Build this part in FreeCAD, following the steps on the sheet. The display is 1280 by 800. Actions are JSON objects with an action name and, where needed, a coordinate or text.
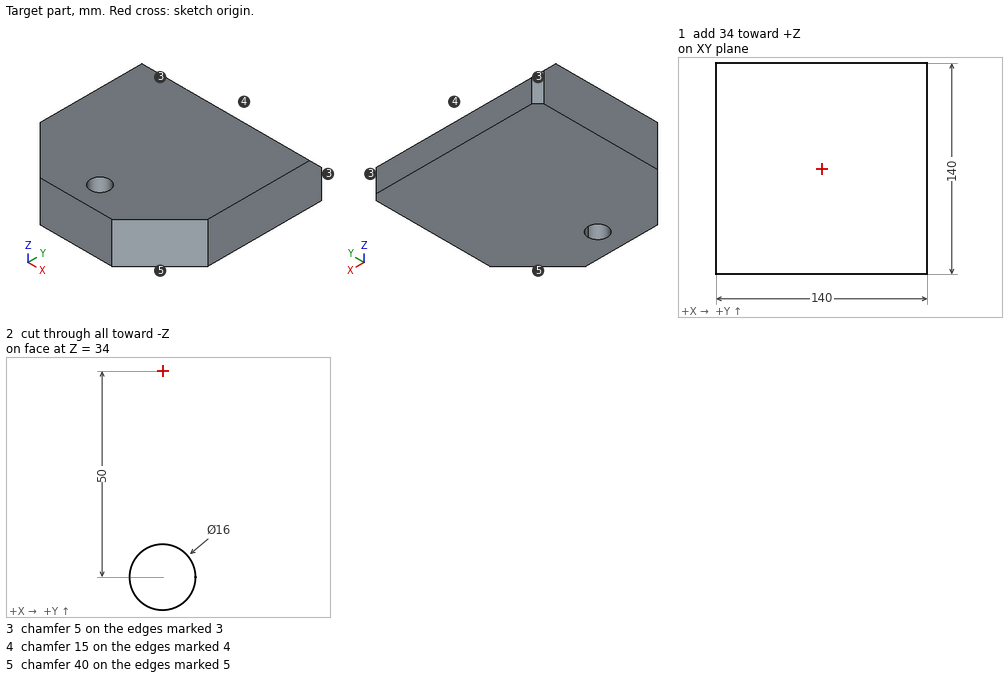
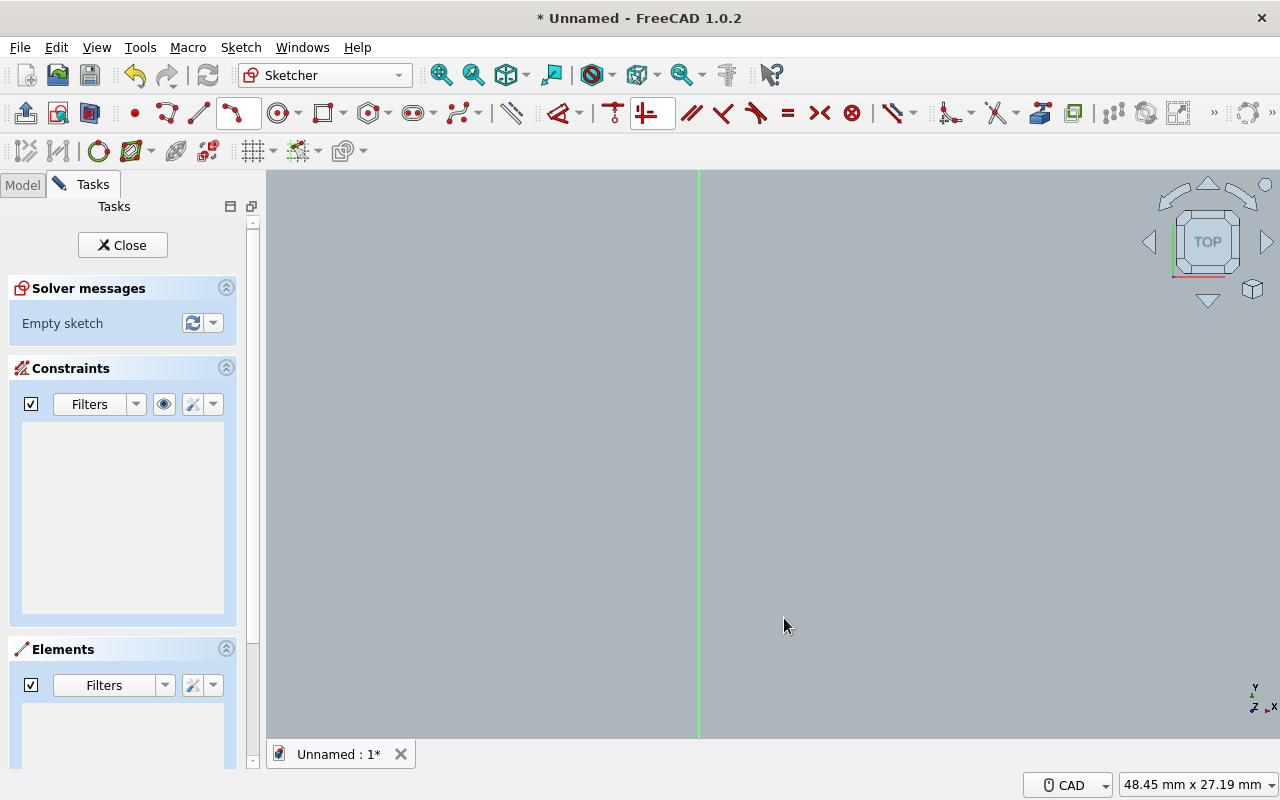
{"action": "left_click", "coordinate": [278, 114]}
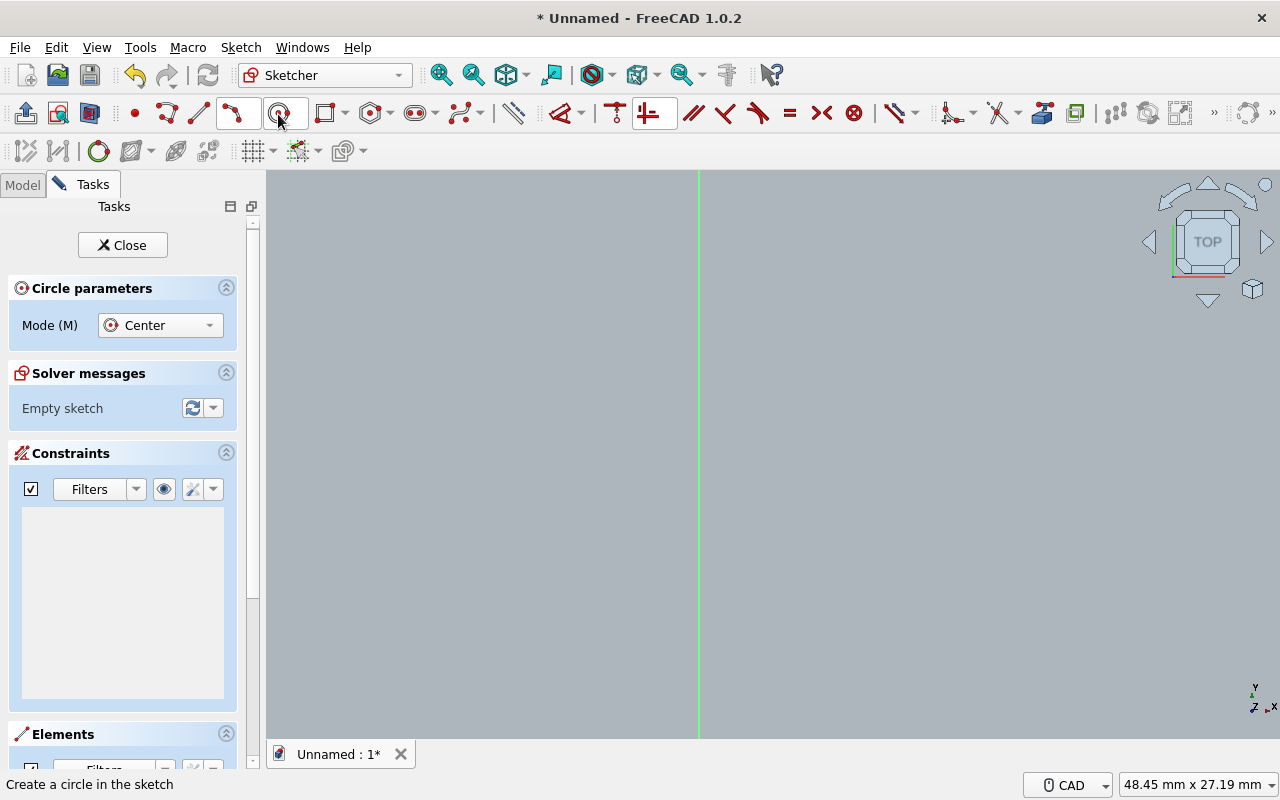
{"action": "left_click", "coordinate": [699, 451]}
{"action": "left_click", "coordinate": [818, 333]}
{"action": "key", "text": "Escape"}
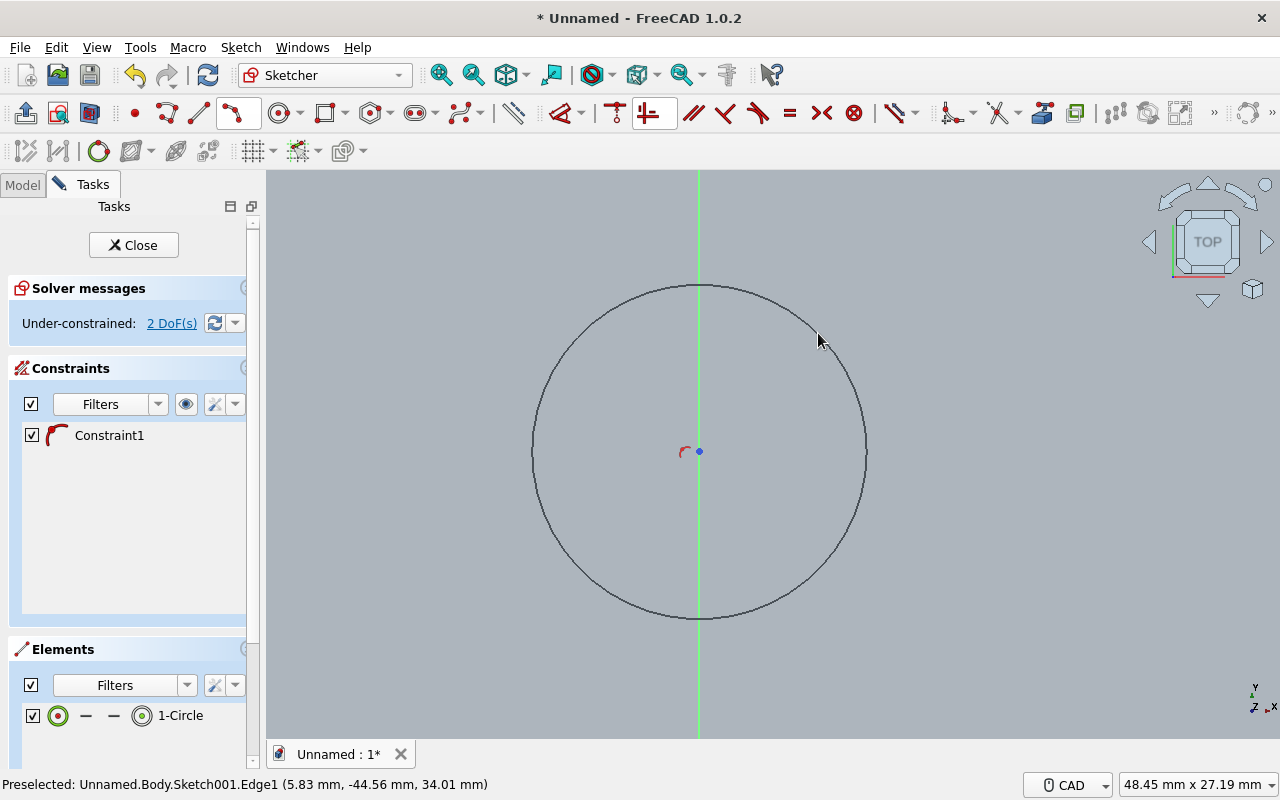
{"action": "left_click", "coordinate": [560, 114]}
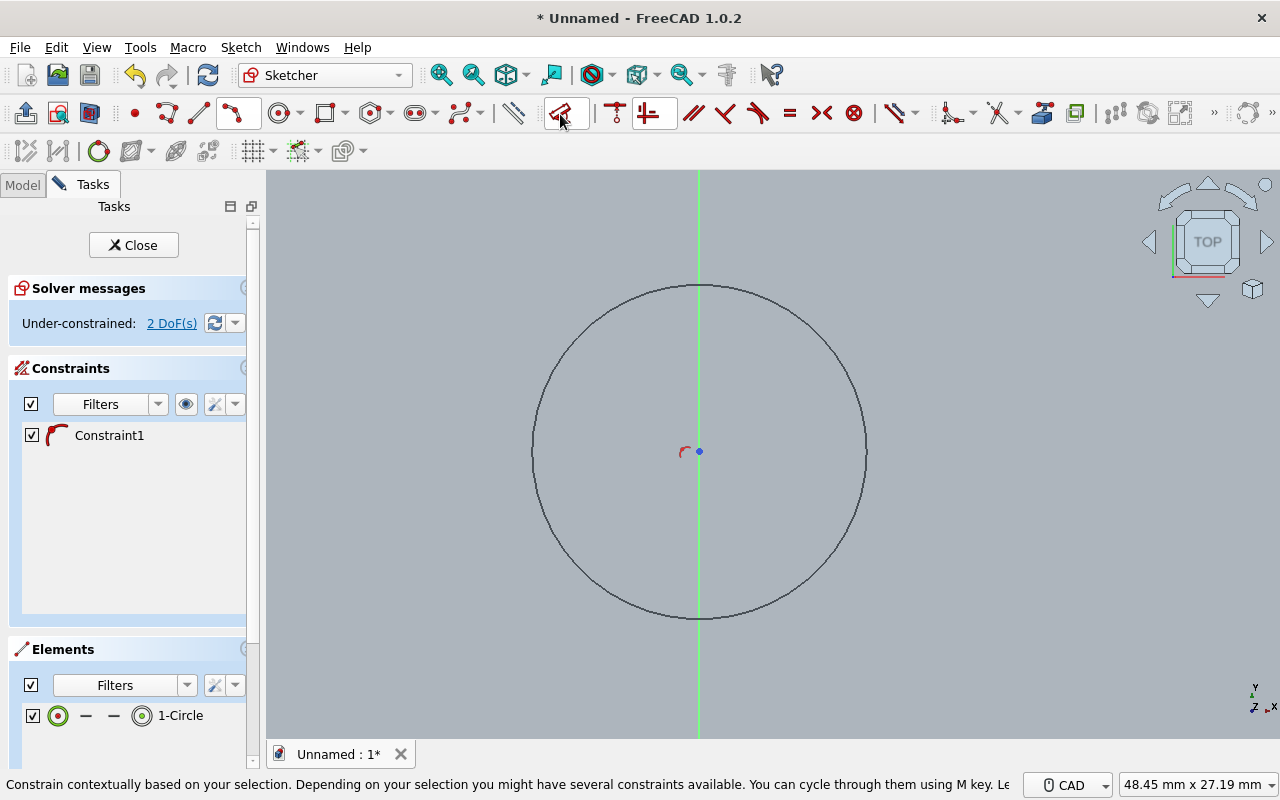
{"action": "left_click", "coordinate": [817, 333]}
{"action": "left_click", "coordinate": [839, 310]}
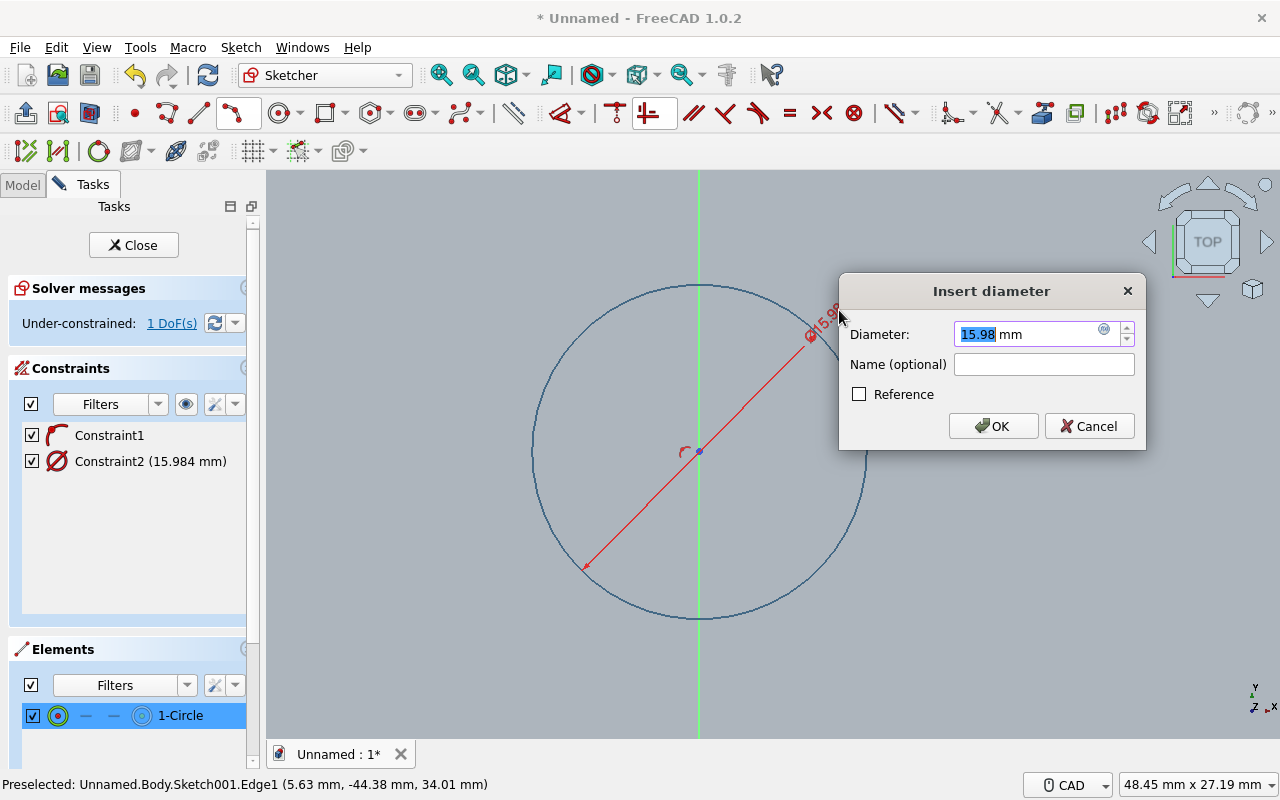
{"action": "type", "text": "16"}
{"action": "key", "text": "Return"}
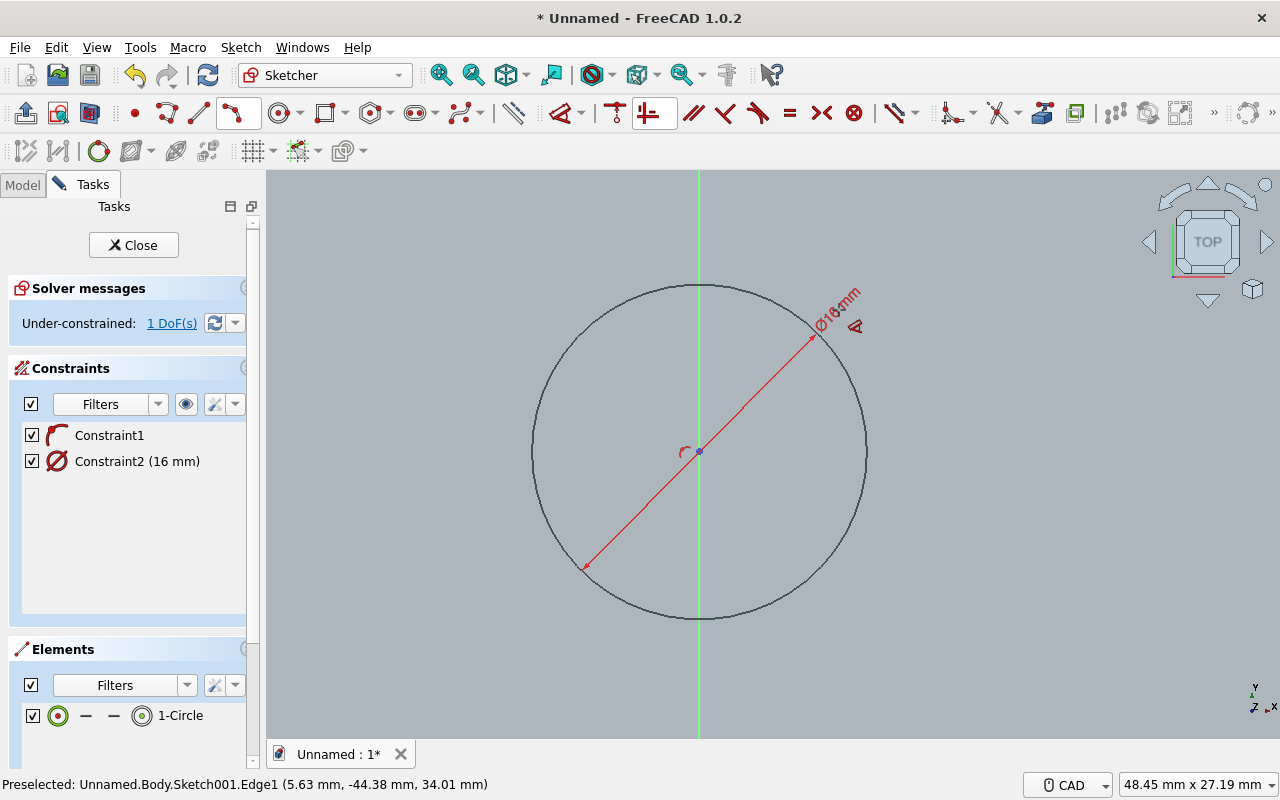
{"action": "left_click", "coordinate": [699, 452]}
{"action": "left_click", "coordinate": [733, 325]}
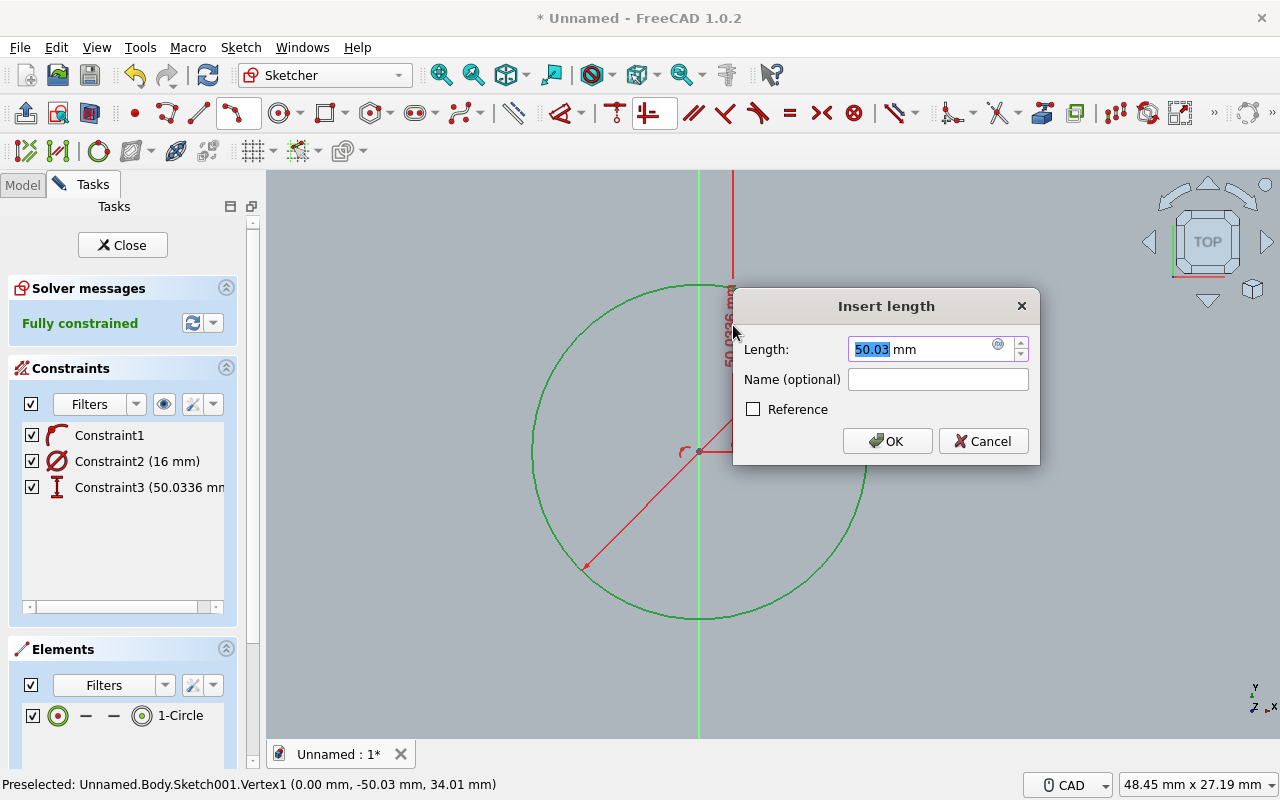
{"action": "type", "text": "50"}
{"action": "key", "text": "Return"}
{"action": "key", "text": "Escape"}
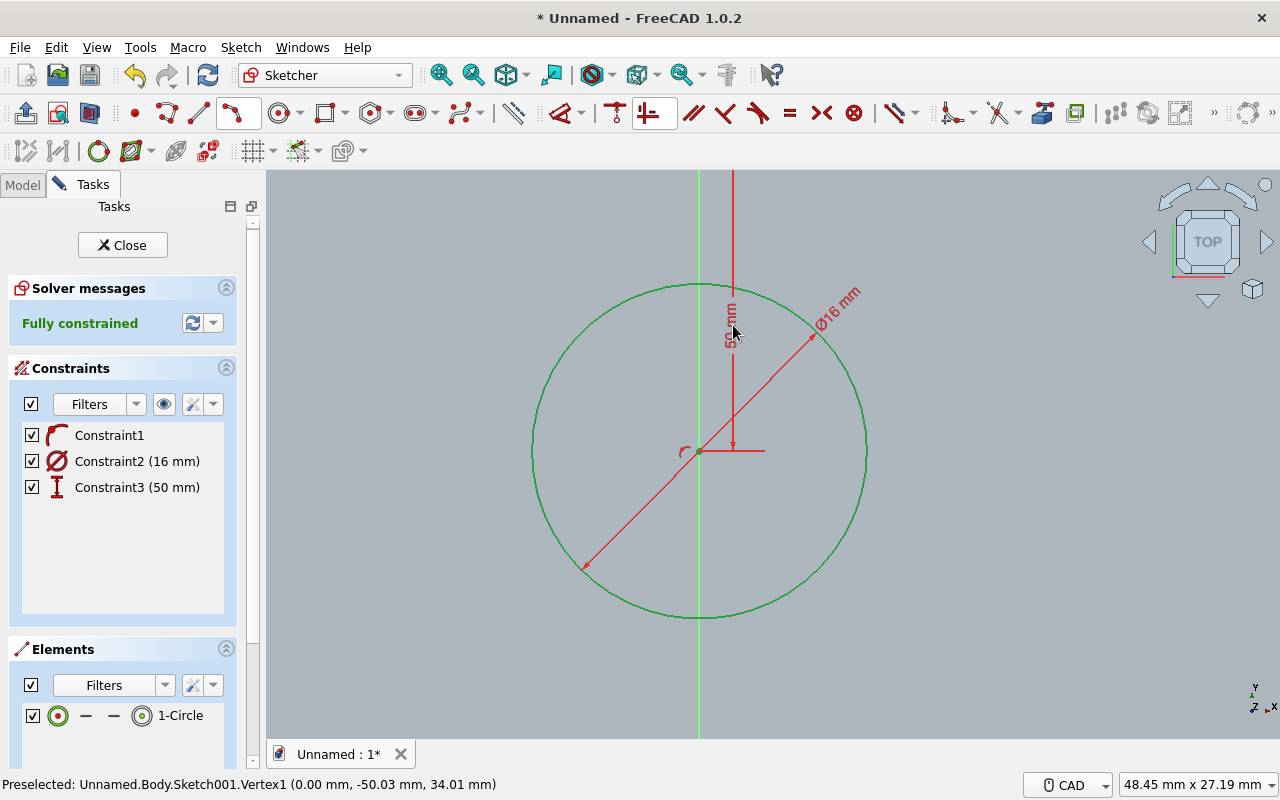
{"action": "left_click", "coordinate": [123, 245]}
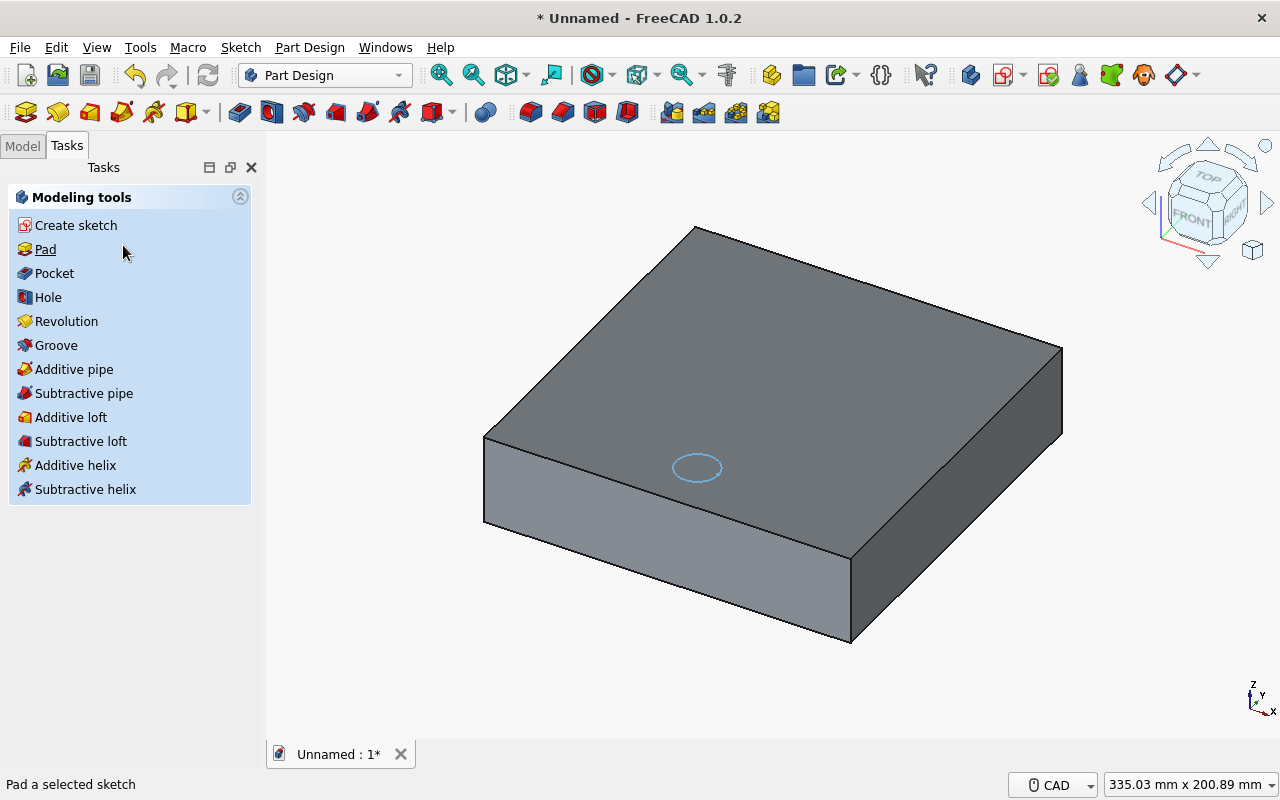
{"action": "left_click", "coordinate": [240, 112]}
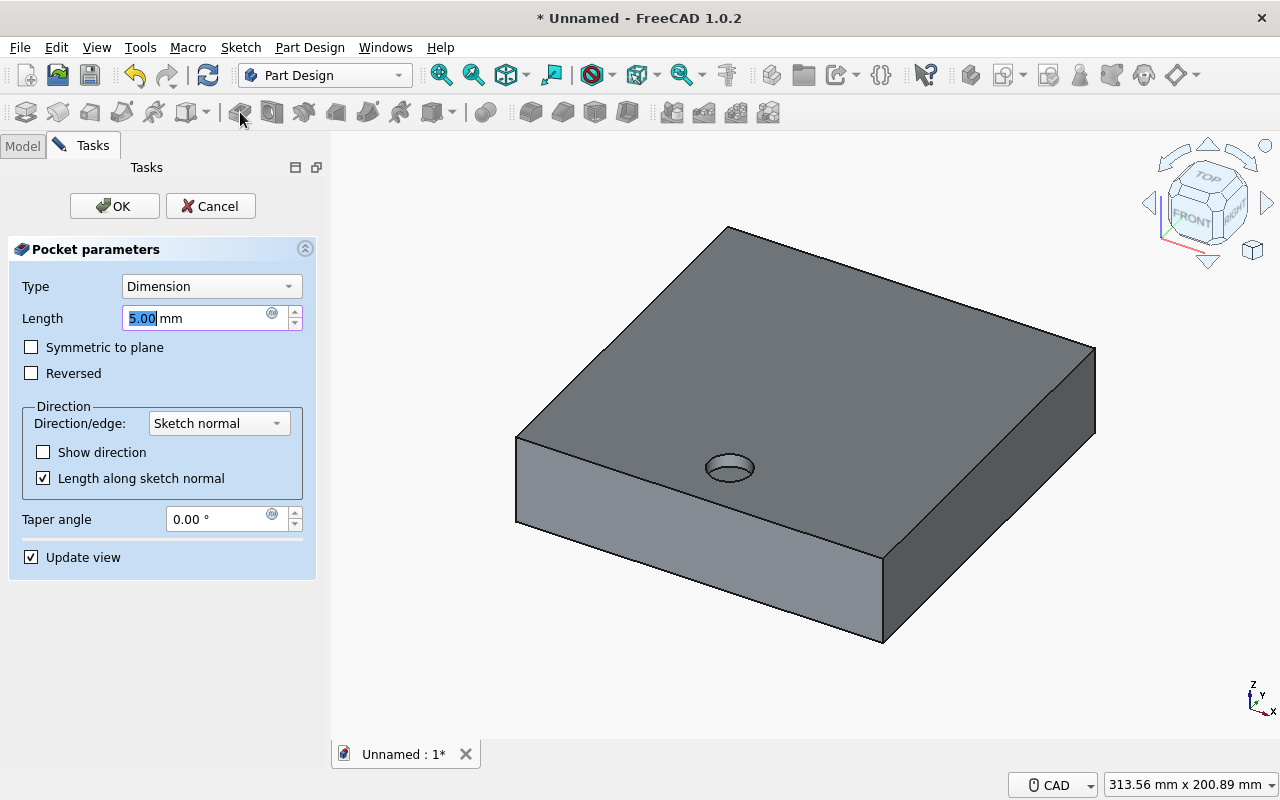
{"action": "left_click", "coordinate": [212, 286]}